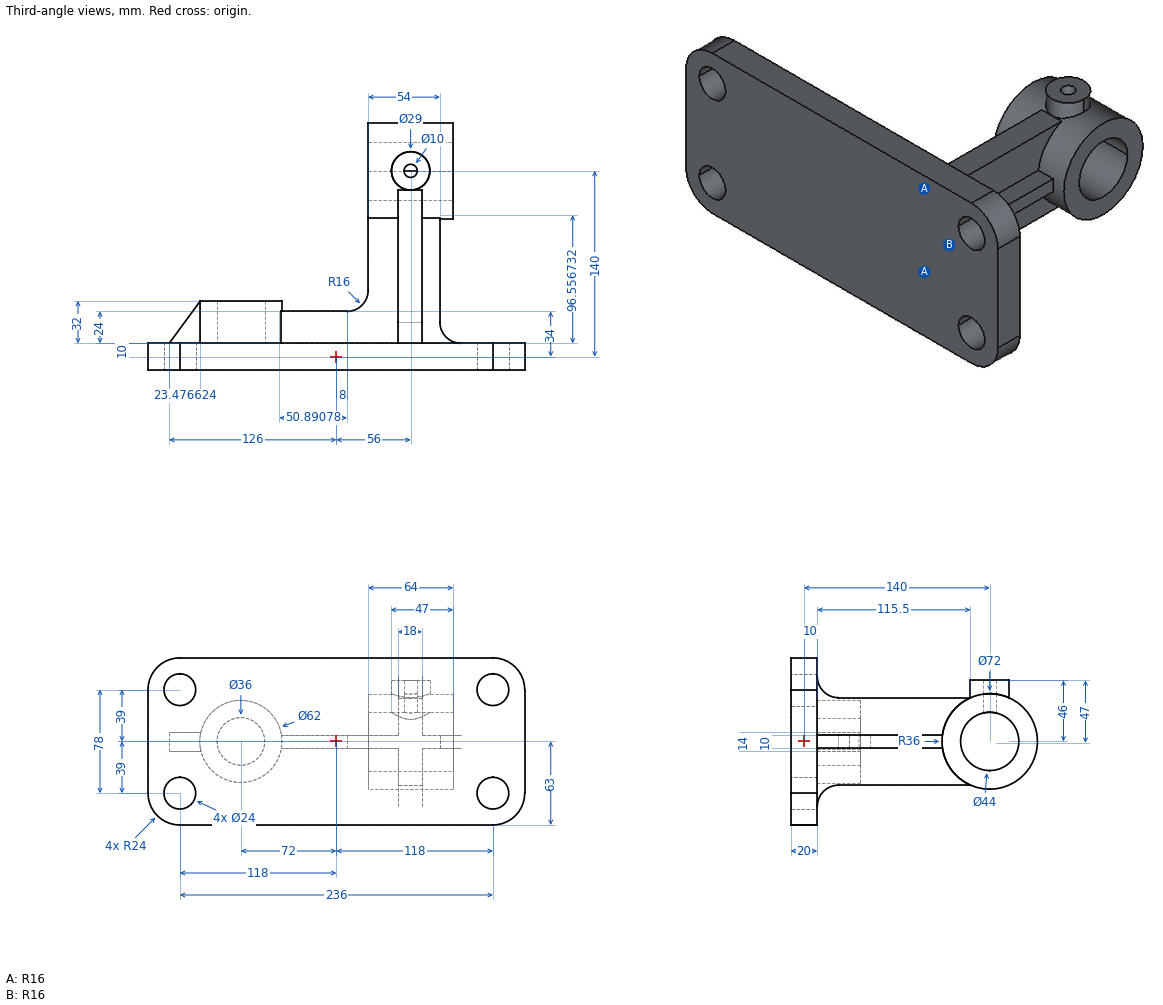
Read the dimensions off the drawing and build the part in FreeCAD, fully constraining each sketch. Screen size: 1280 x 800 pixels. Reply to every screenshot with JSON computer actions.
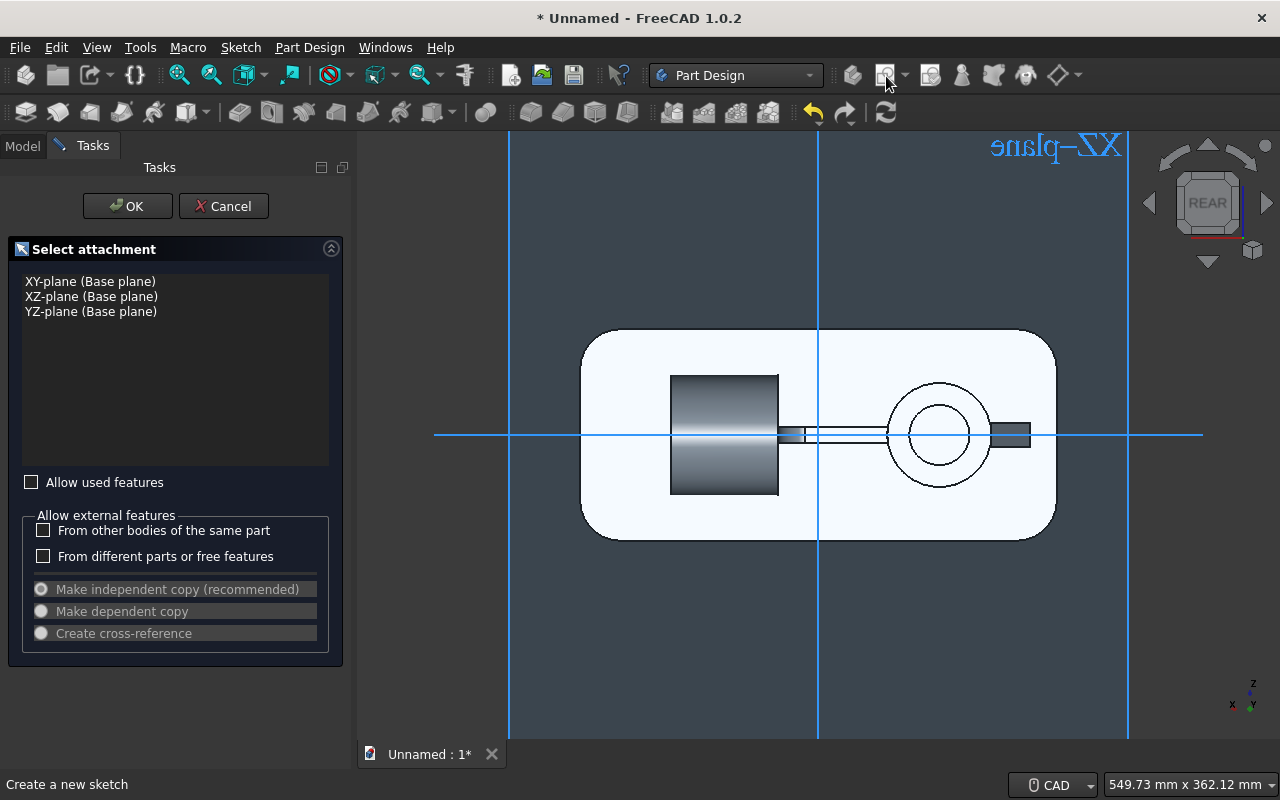
{"action": "left_click", "coordinate": [82, 282]}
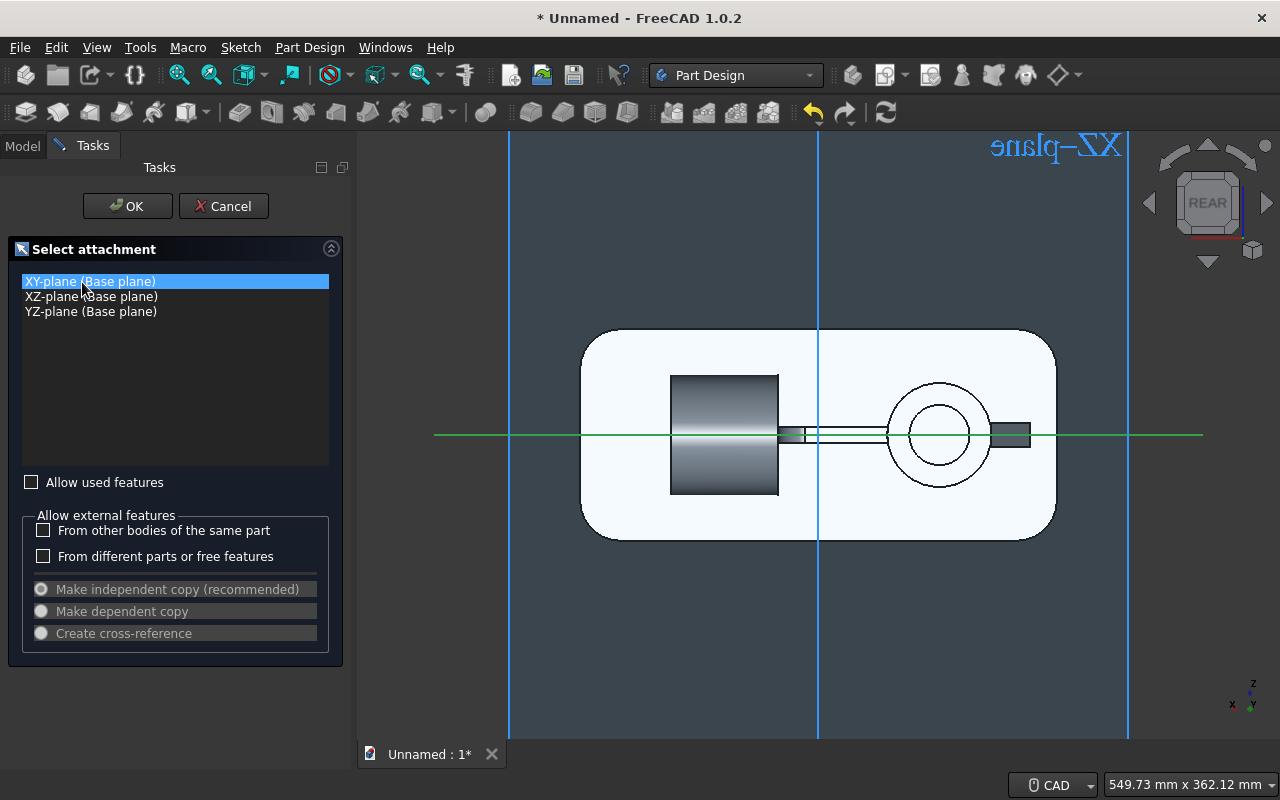
{"action": "left_click", "coordinate": [128, 206]}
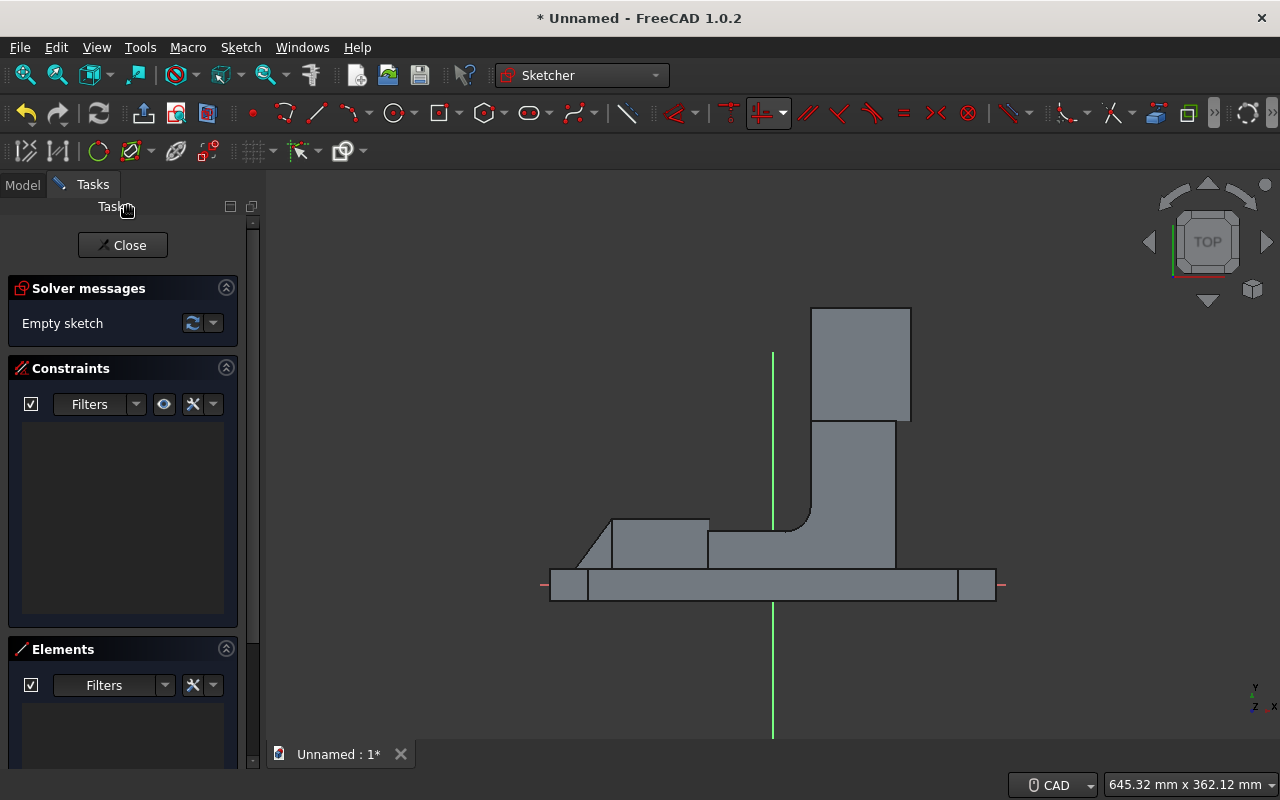
{"action": "left_click", "coordinate": [208, 114]}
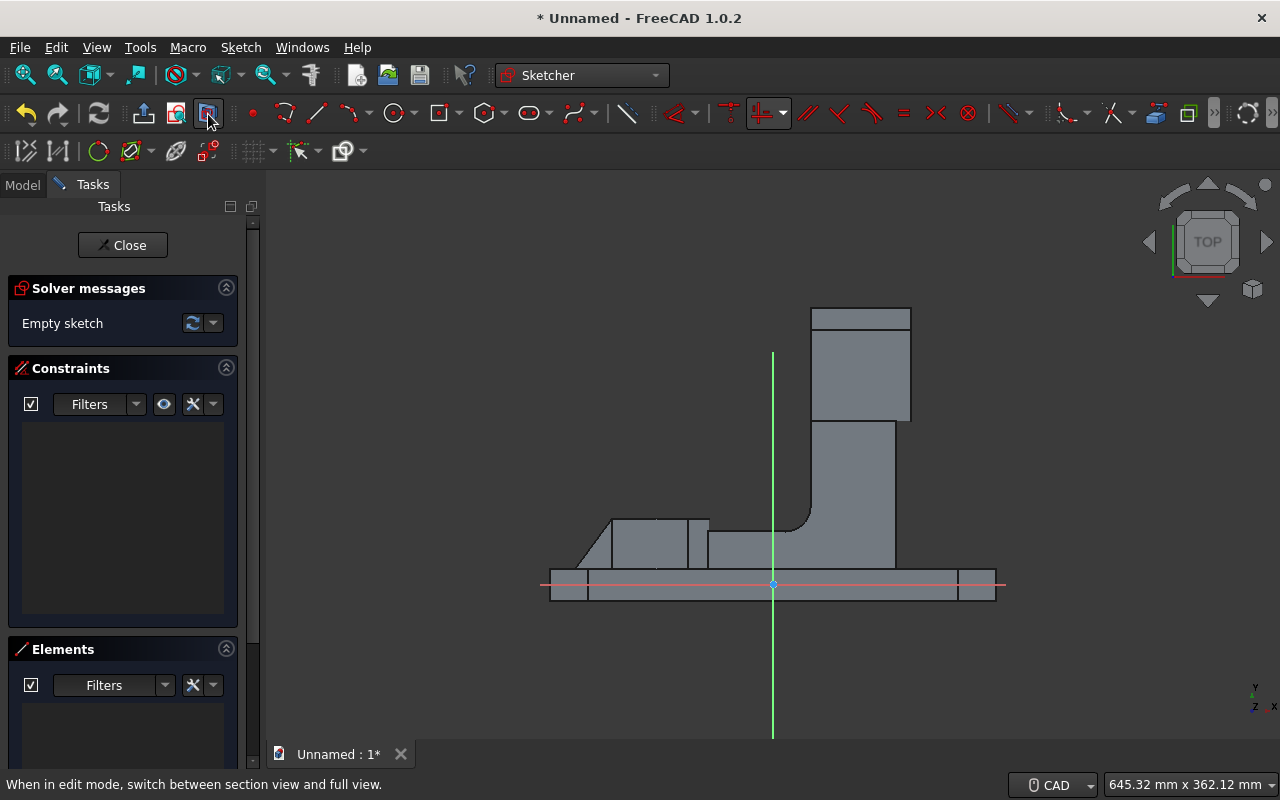
{"action": "scroll", "coordinate": [885, 351], "scroll_direction": "up", "scroll_amount": 10}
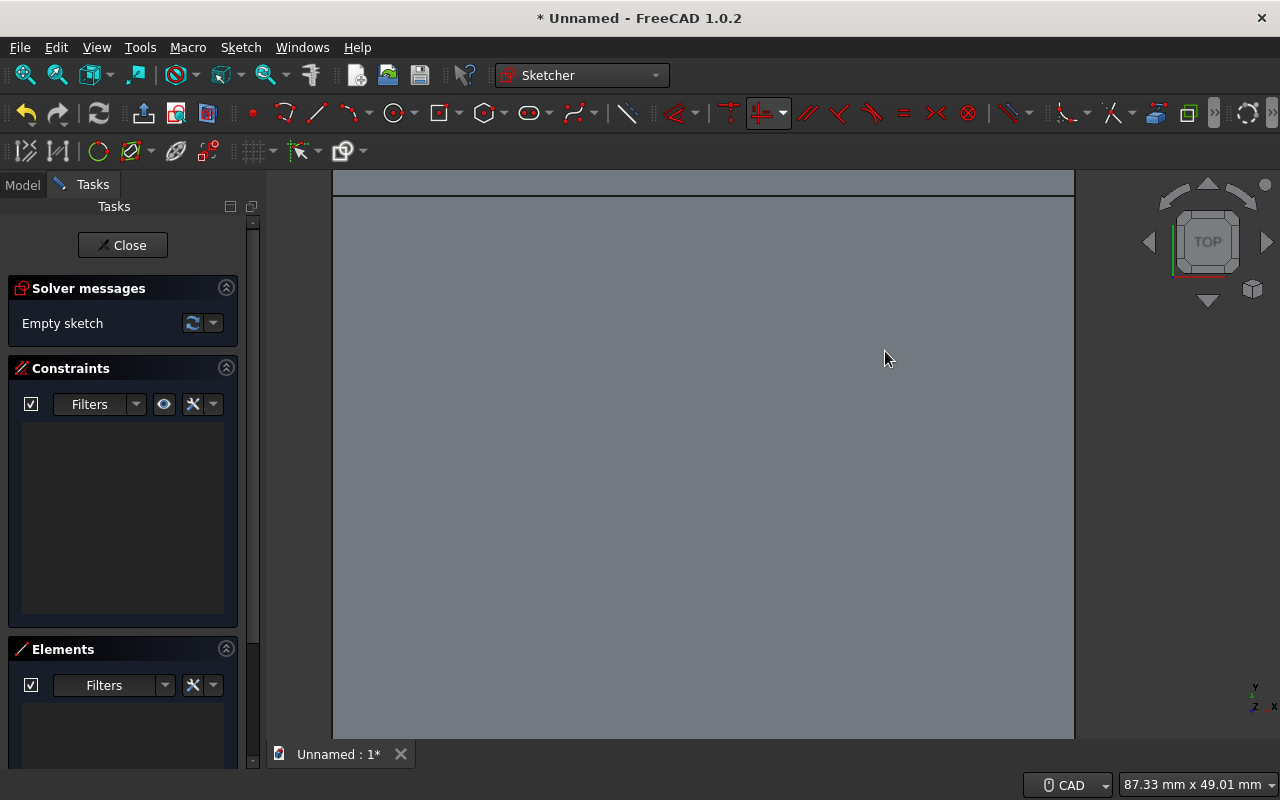
{"action": "left_click", "coordinate": [394, 114]}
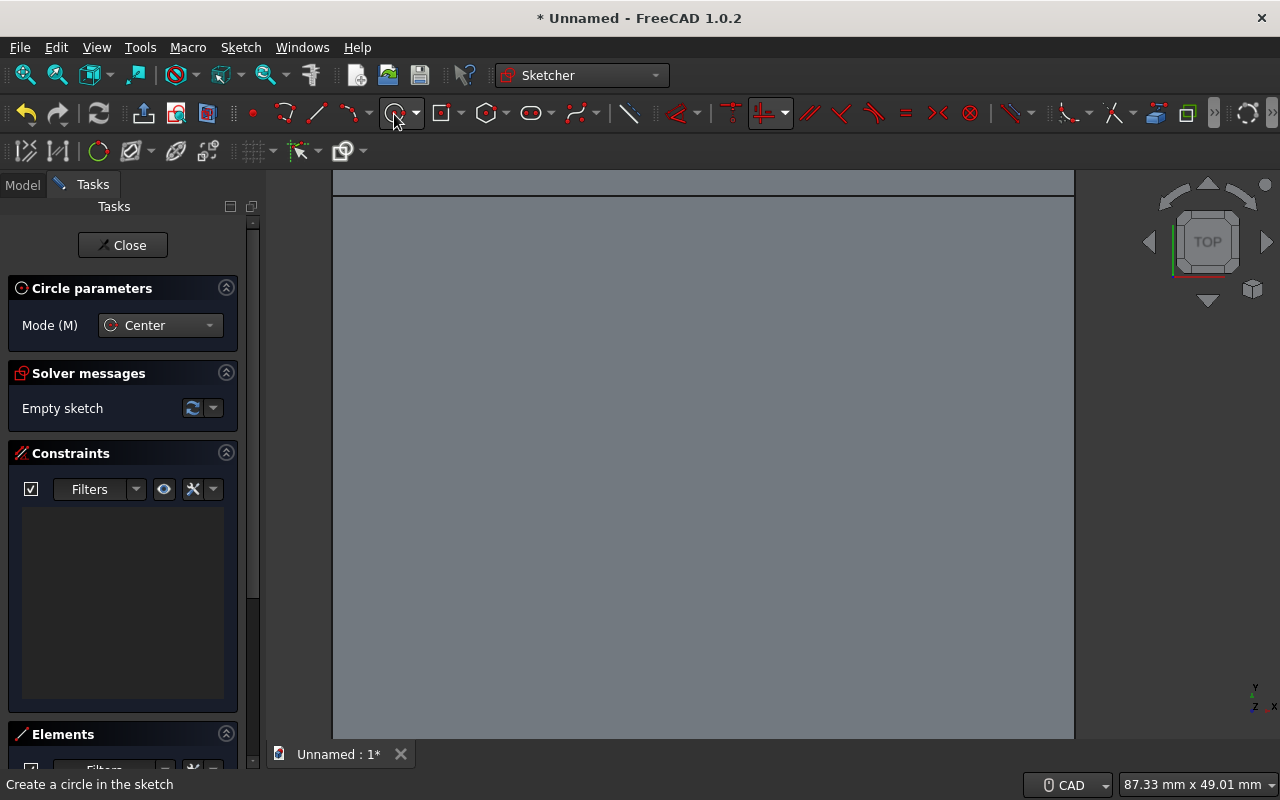
{"action": "left_click", "coordinate": [704, 452]}
{"action": "mouse_move", "coordinate": [823, 333]}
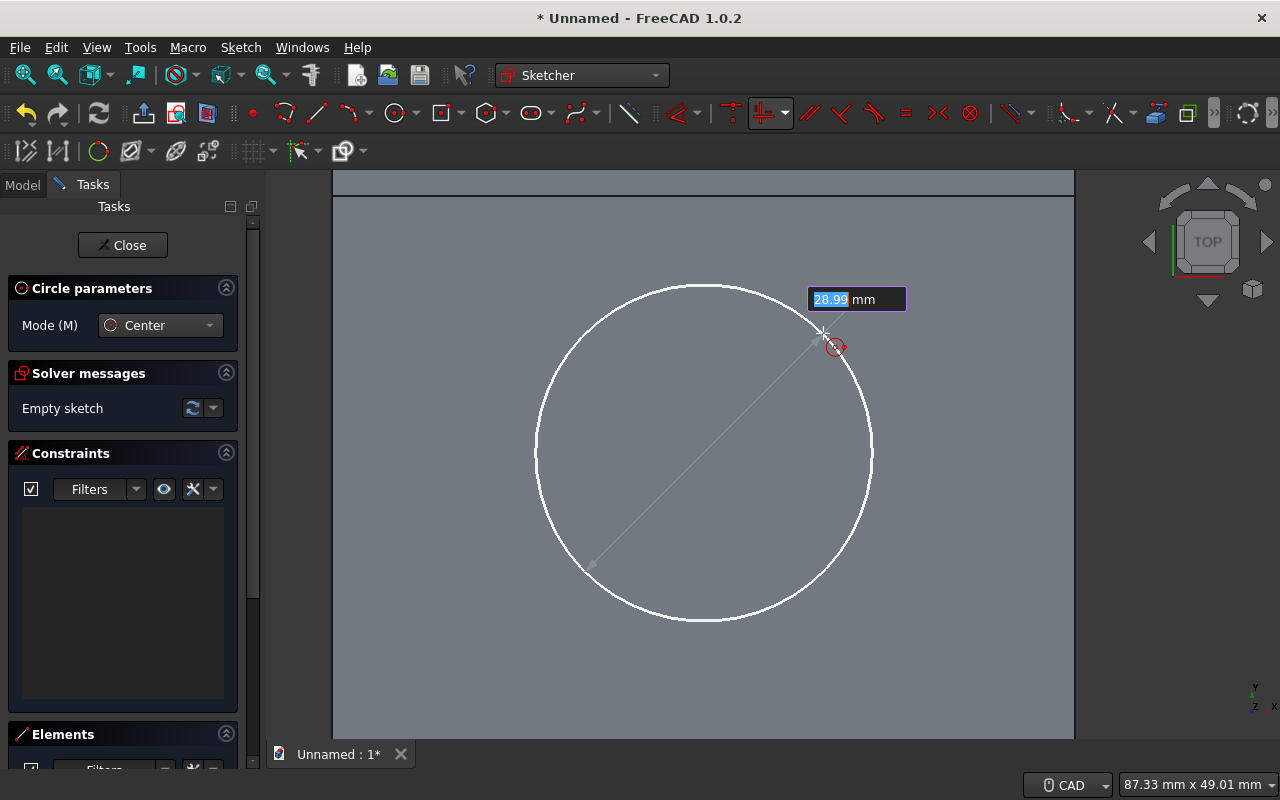
{"action": "type", "text": "29"}
{"action": "key", "text": "Return"}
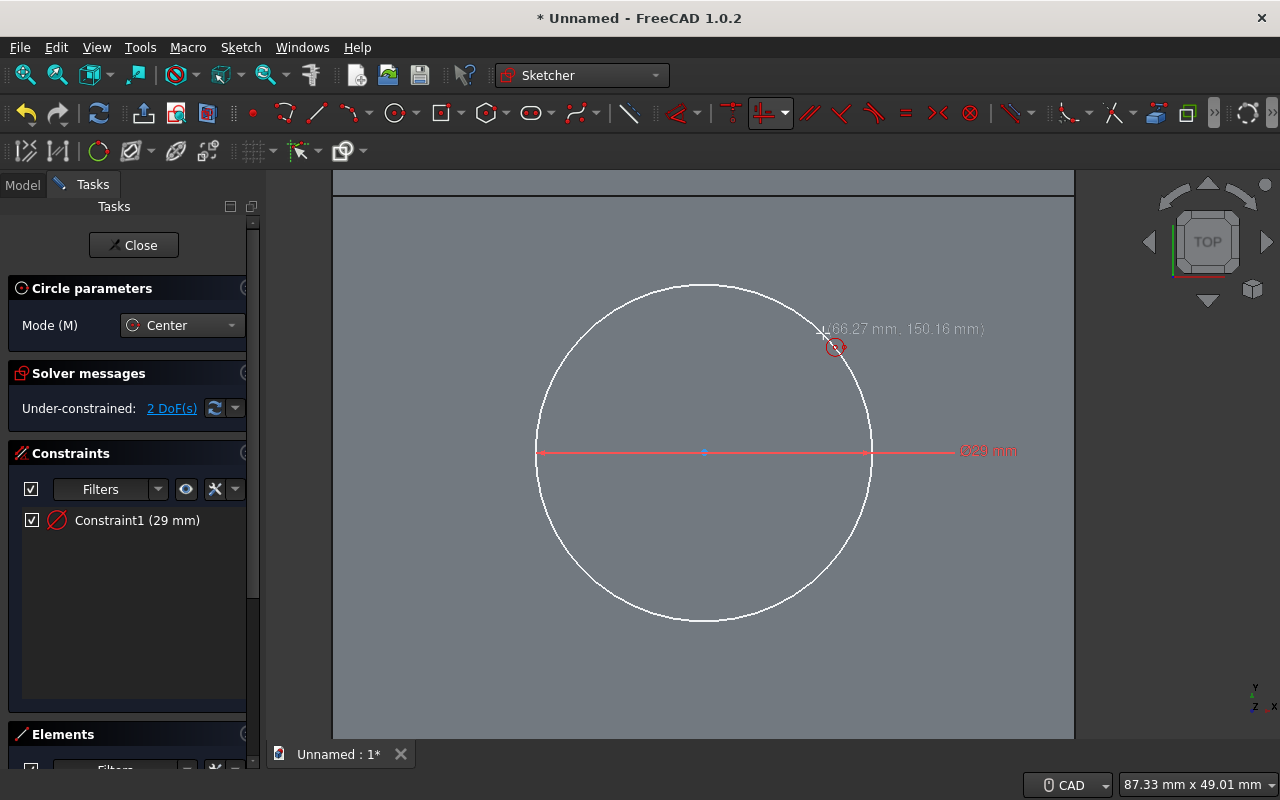
{"action": "left_click", "coordinate": [704, 453]}
{"action": "mouse_move", "coordinate": [745, 411]}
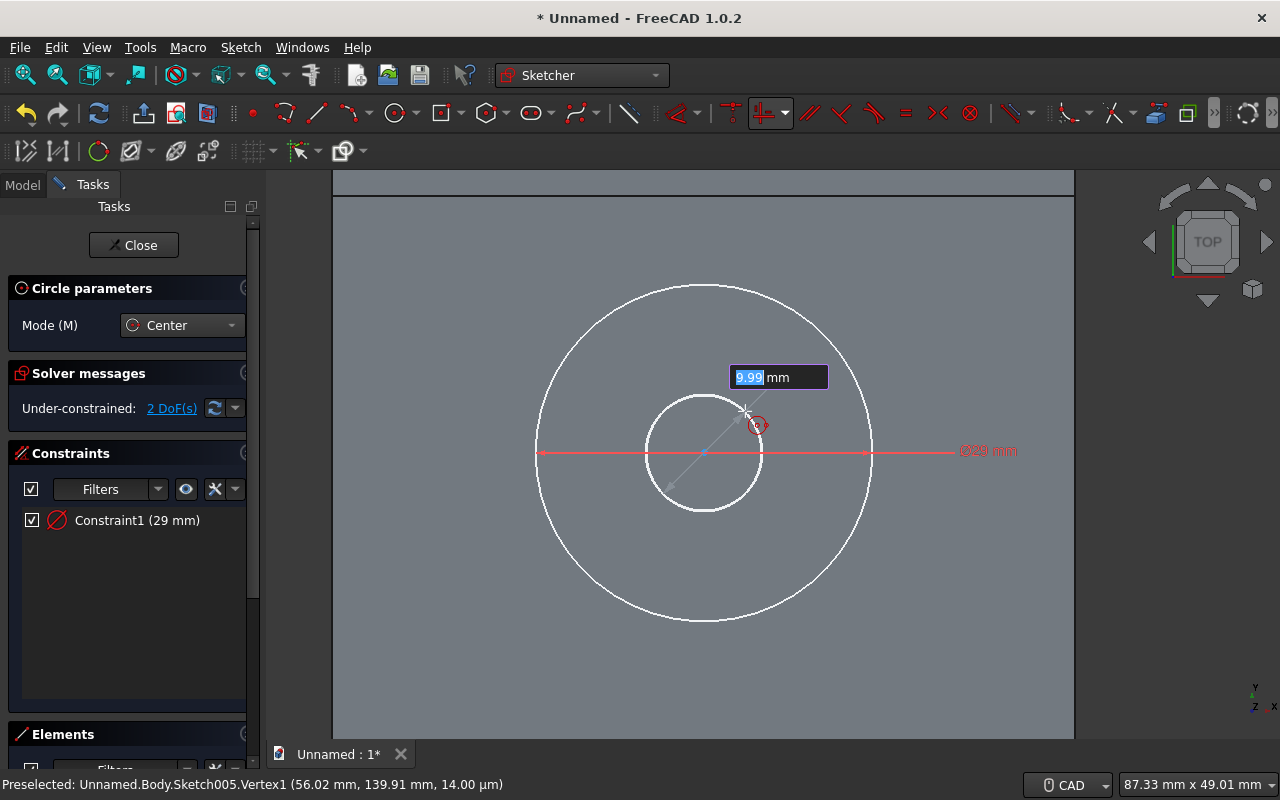
{"action": "type", "text": "10"}
{"action": "key", "text": "Return"}
{"action": "key", "text": "Escape"}